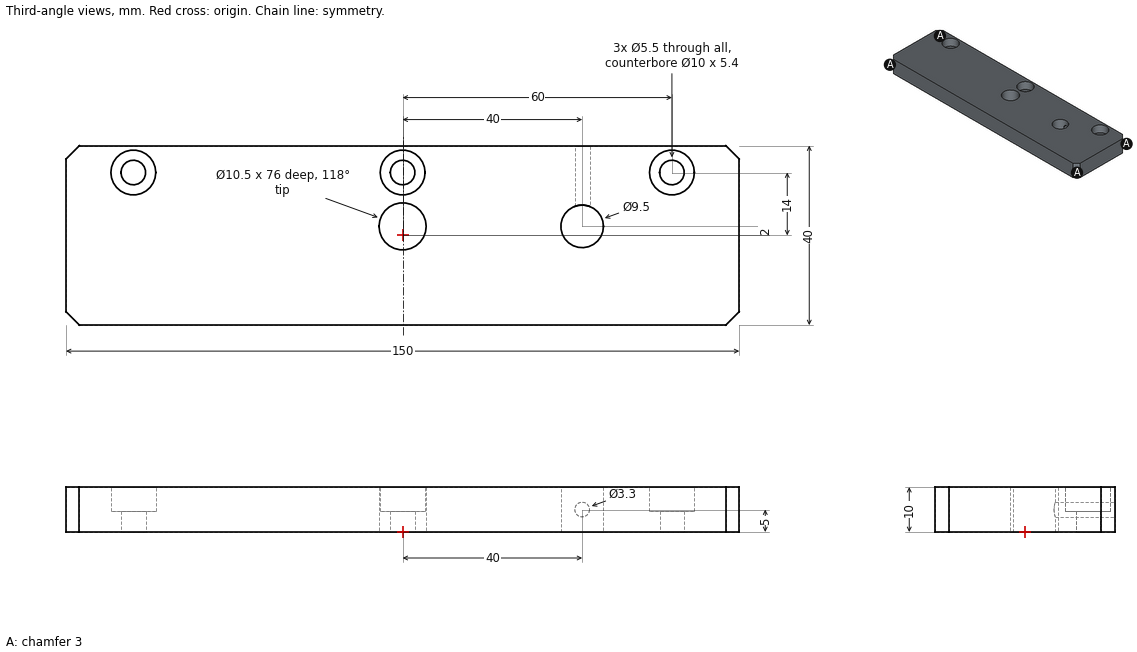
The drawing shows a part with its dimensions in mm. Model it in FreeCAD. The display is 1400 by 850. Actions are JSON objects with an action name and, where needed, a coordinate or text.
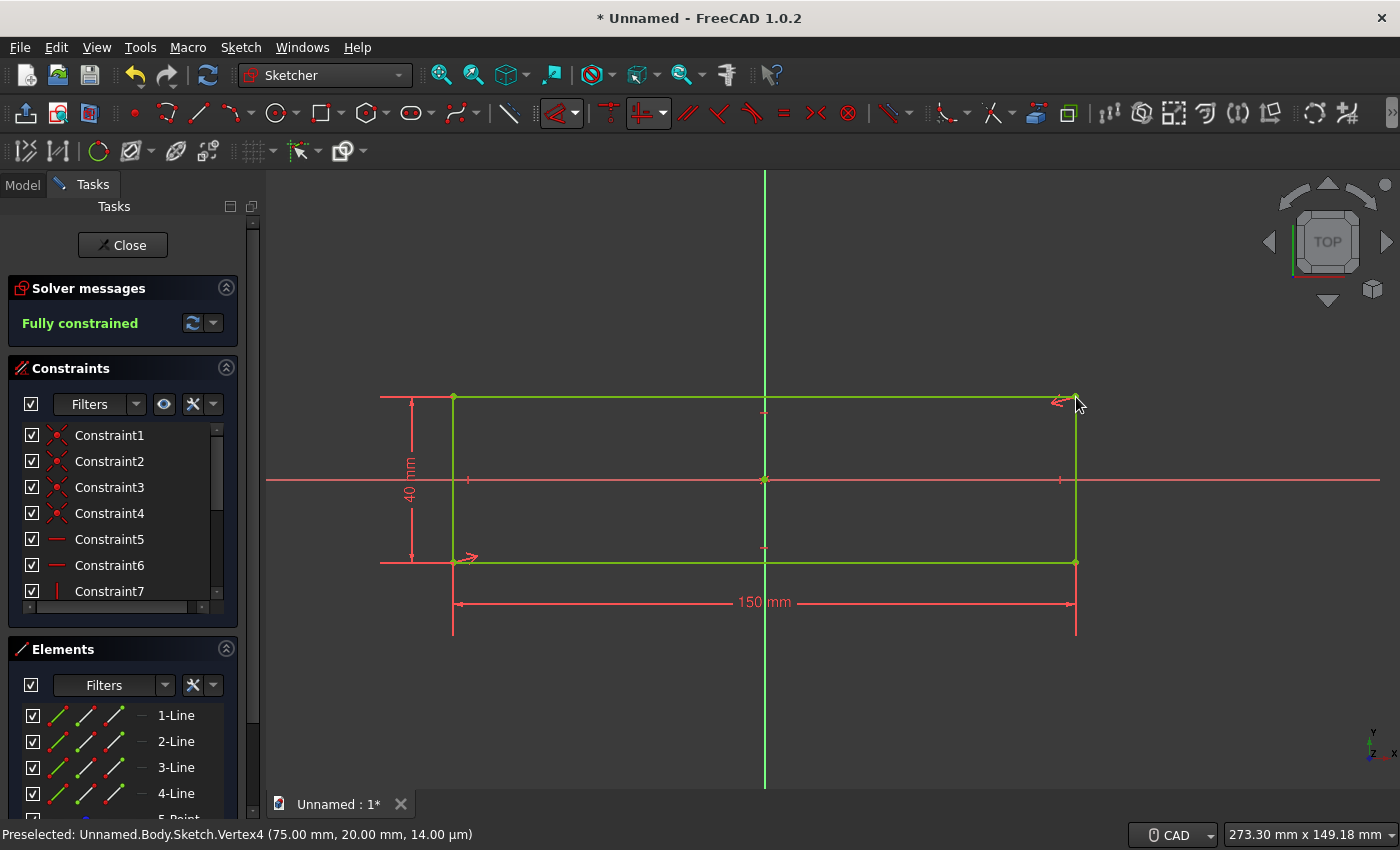
{"action": "left_click", "coordinate": [123, 245]}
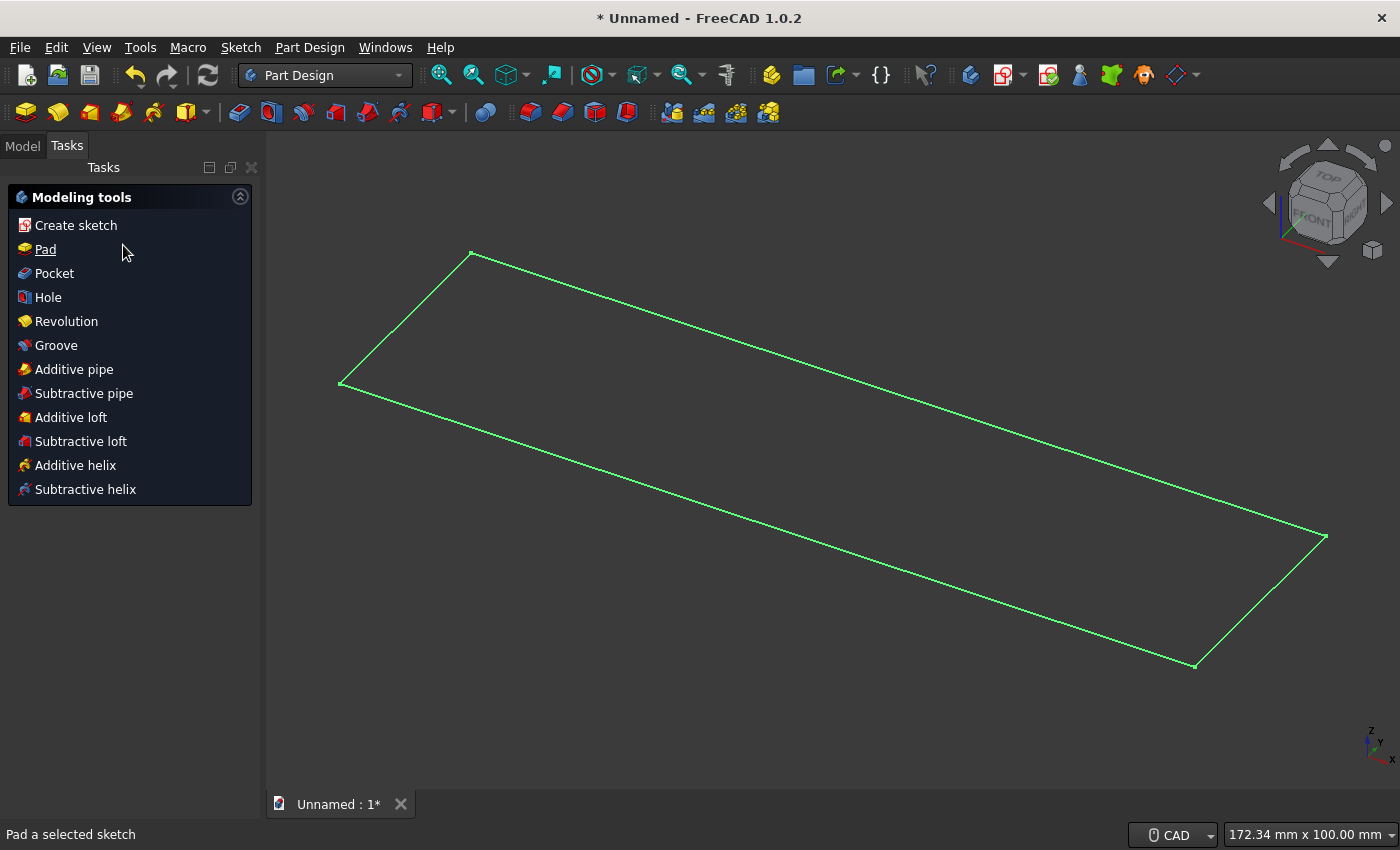
{"action": "left_click", "coordinate": [26, 112]}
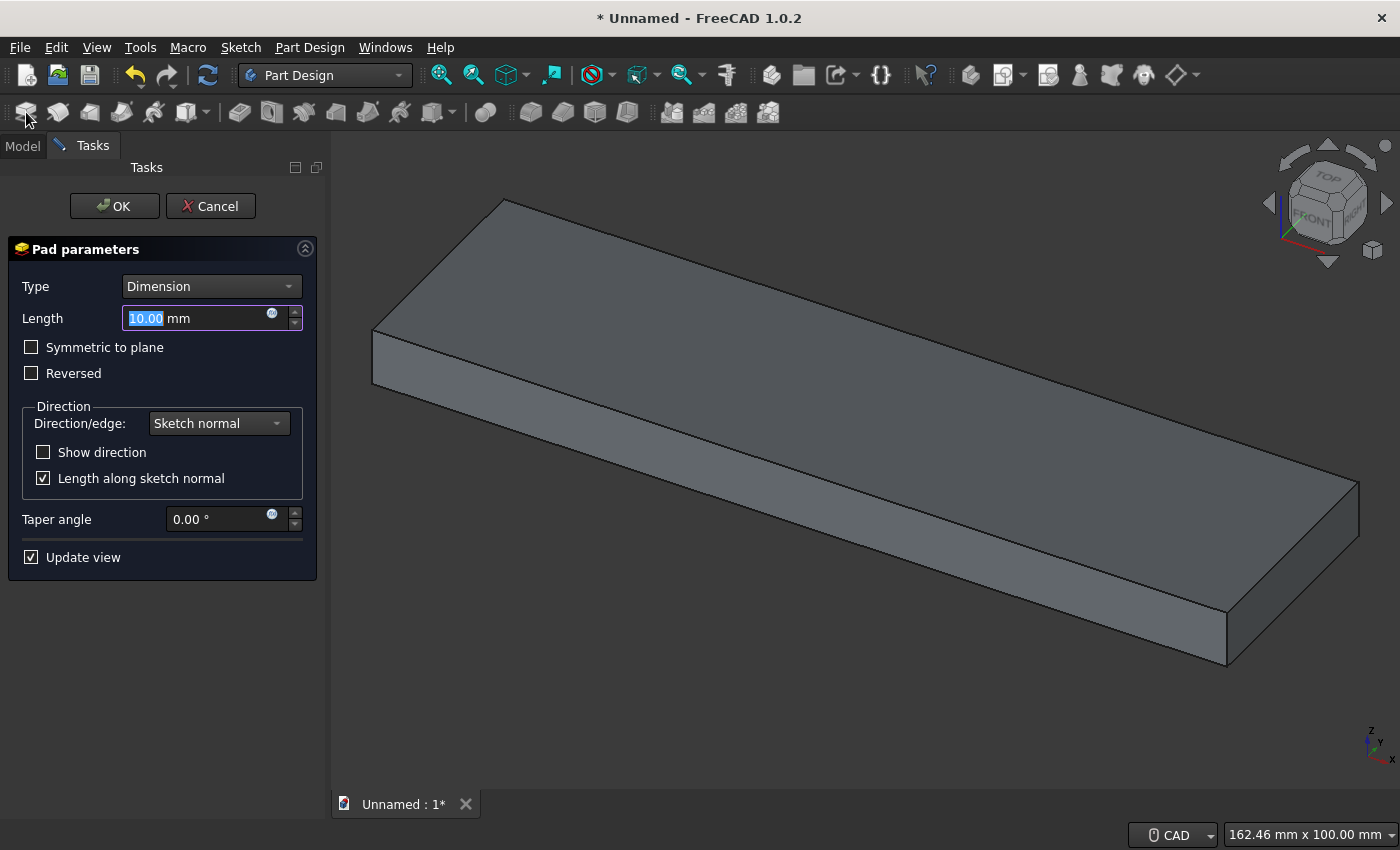
{"action": "type", "text": "10"}
{"action": "key", "text": "Tab"}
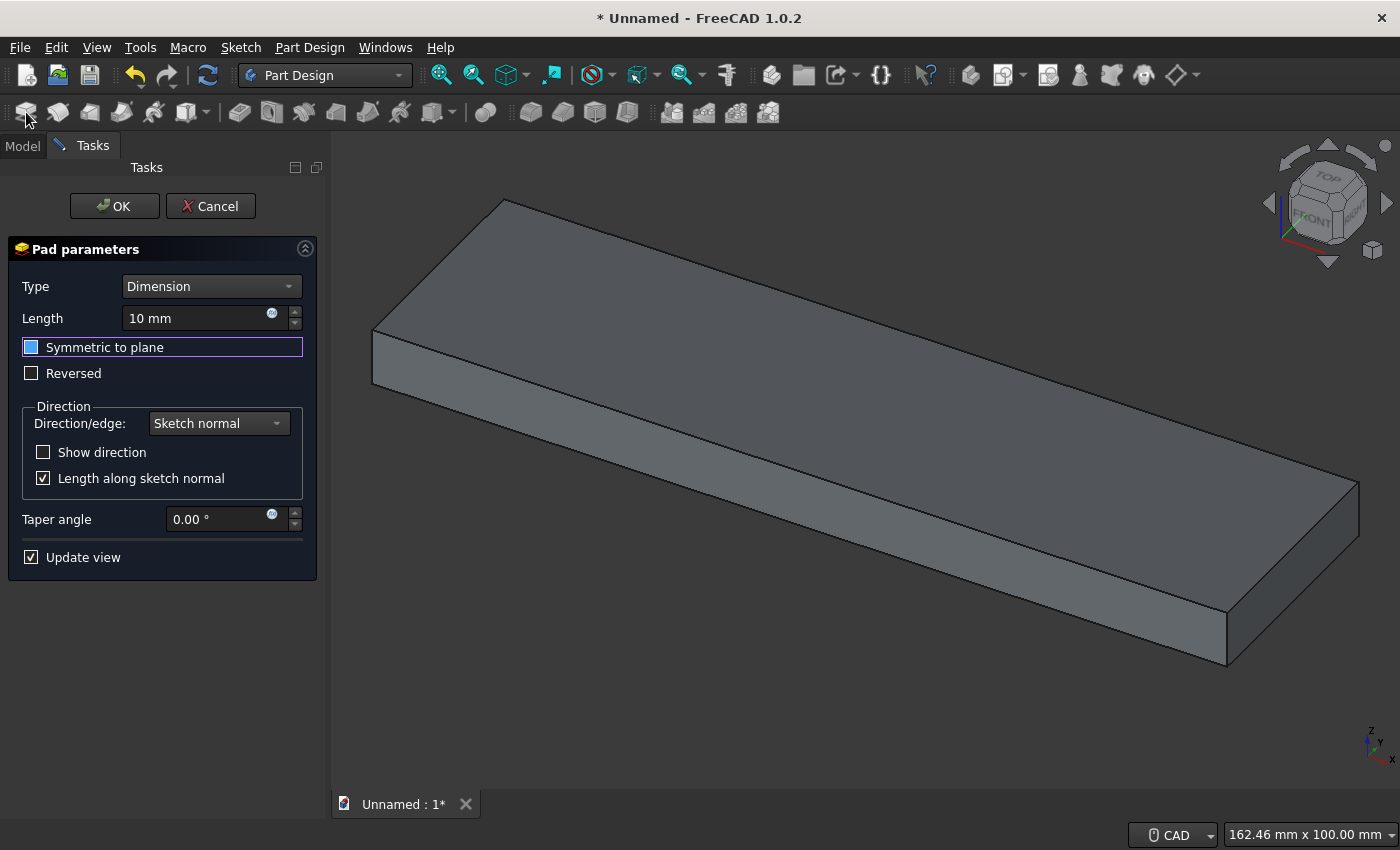
{"action": "left_click", "coordinate": [115, 206]}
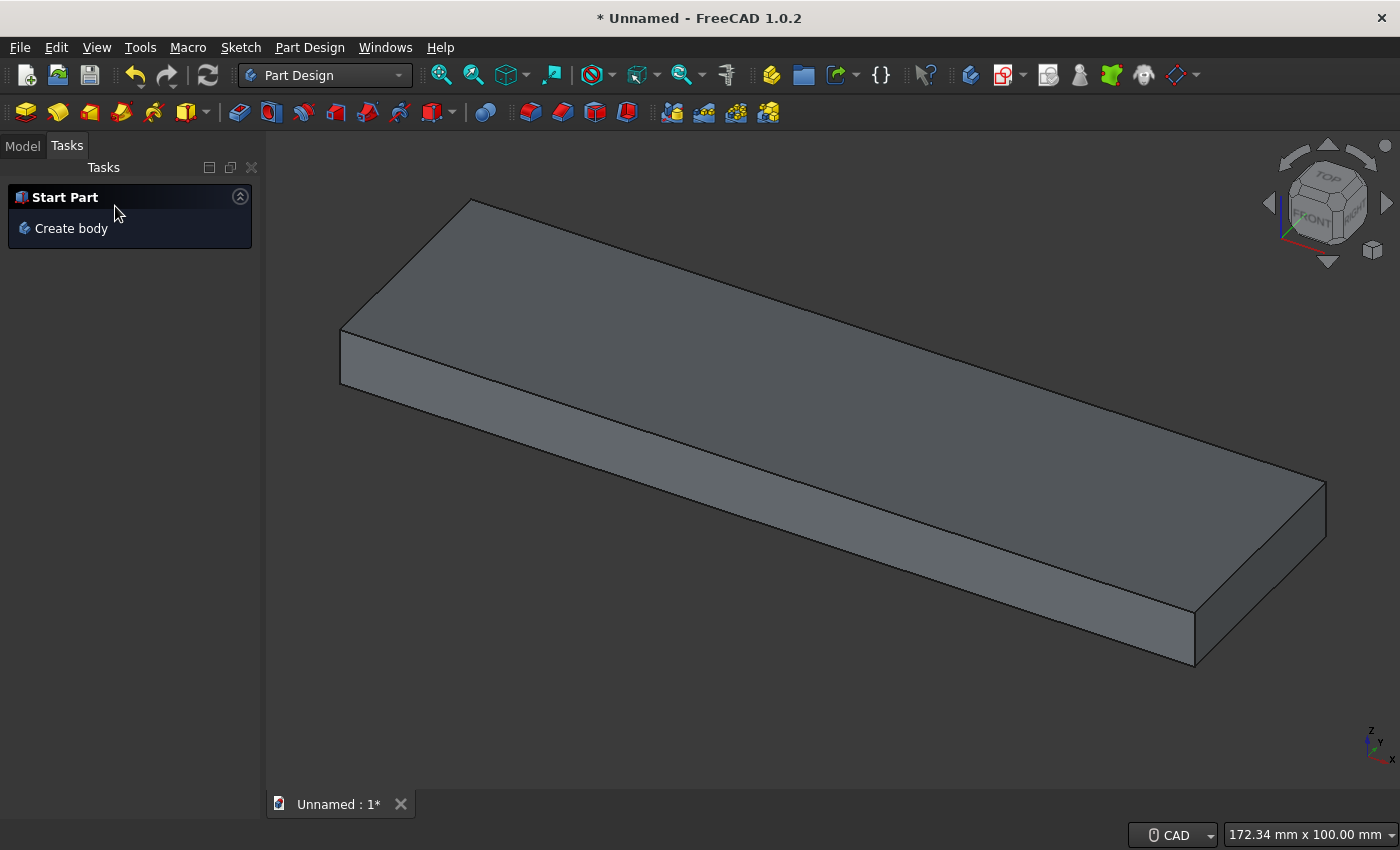
{"action": "left_click", "coordinate": [1077, 486]}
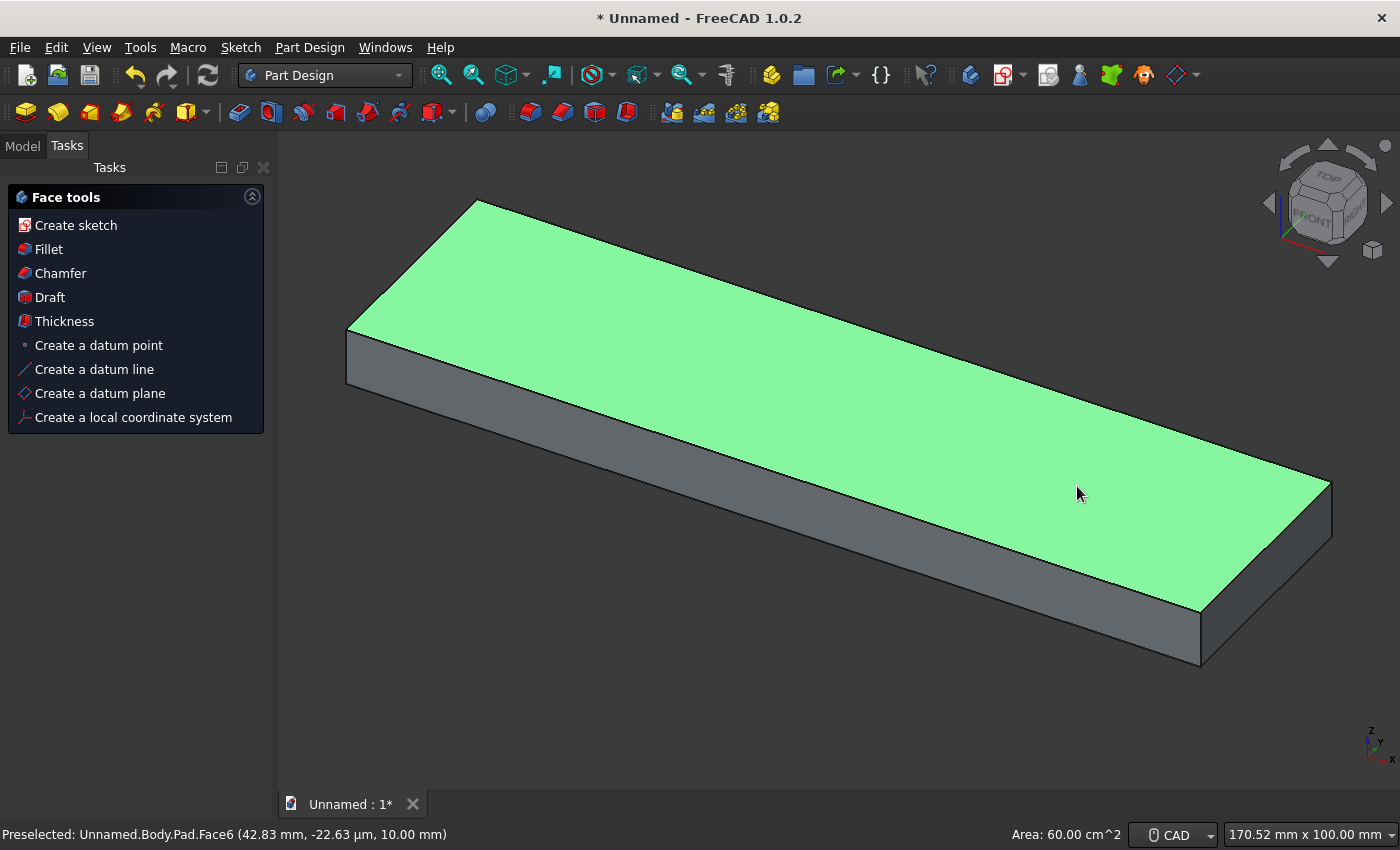
{"action": "left_click", "coordinate": [1004, 76]}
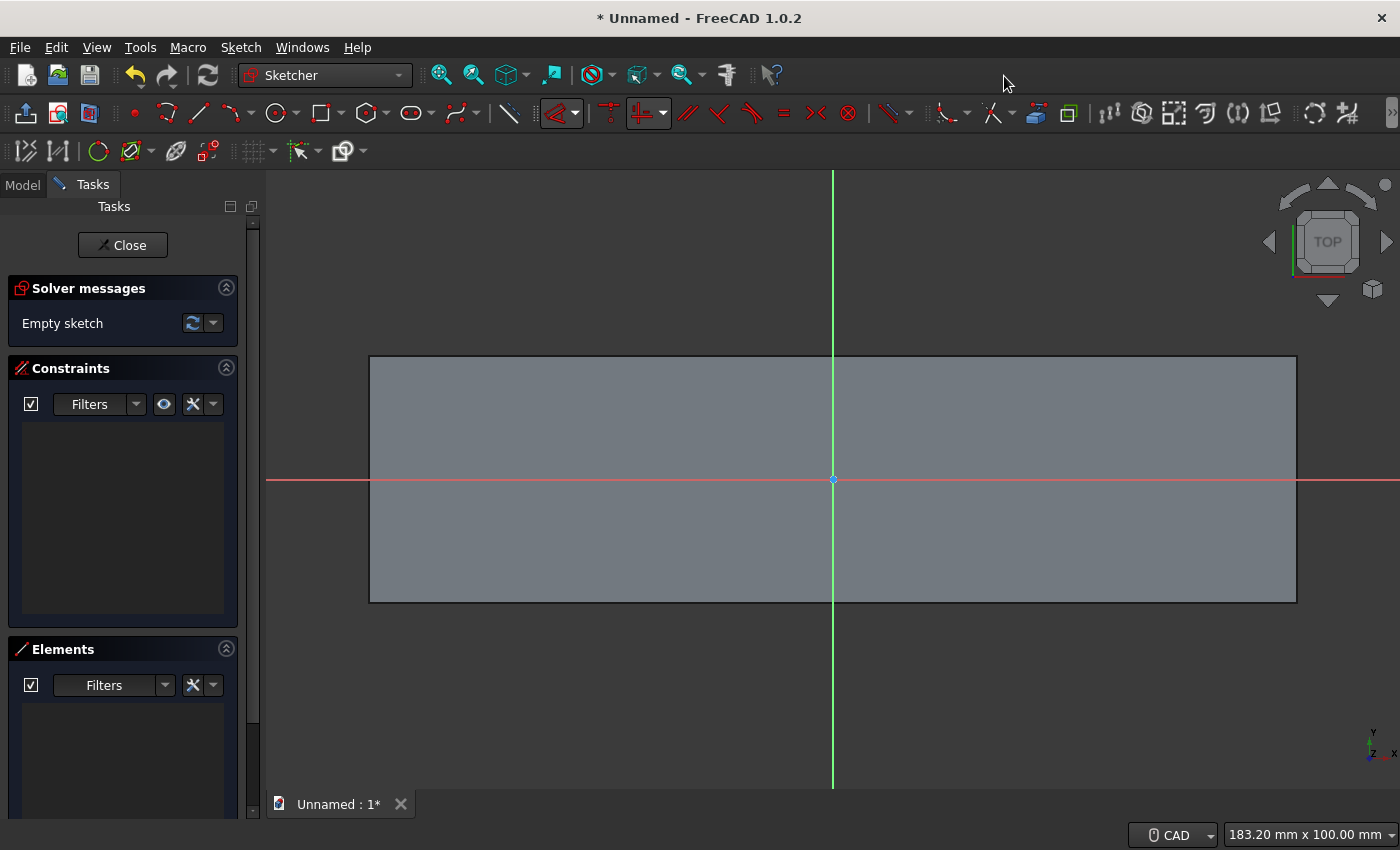
{"action": "scroll", "coordinate": [1130, 465], "scroll_direction": "up", "scroll_amount": 10}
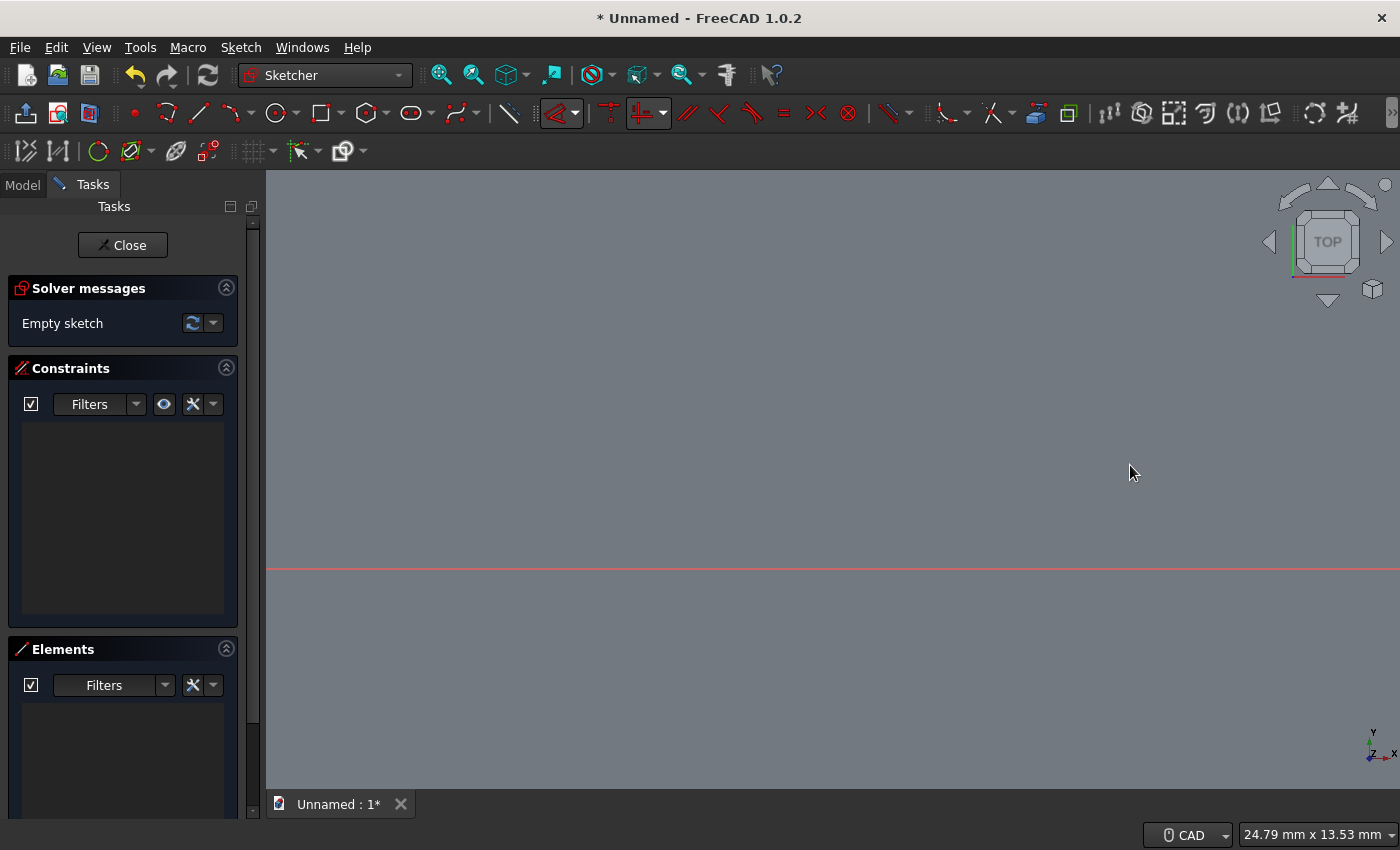
{"action": "left_click", "coordinate": [276, 114]}